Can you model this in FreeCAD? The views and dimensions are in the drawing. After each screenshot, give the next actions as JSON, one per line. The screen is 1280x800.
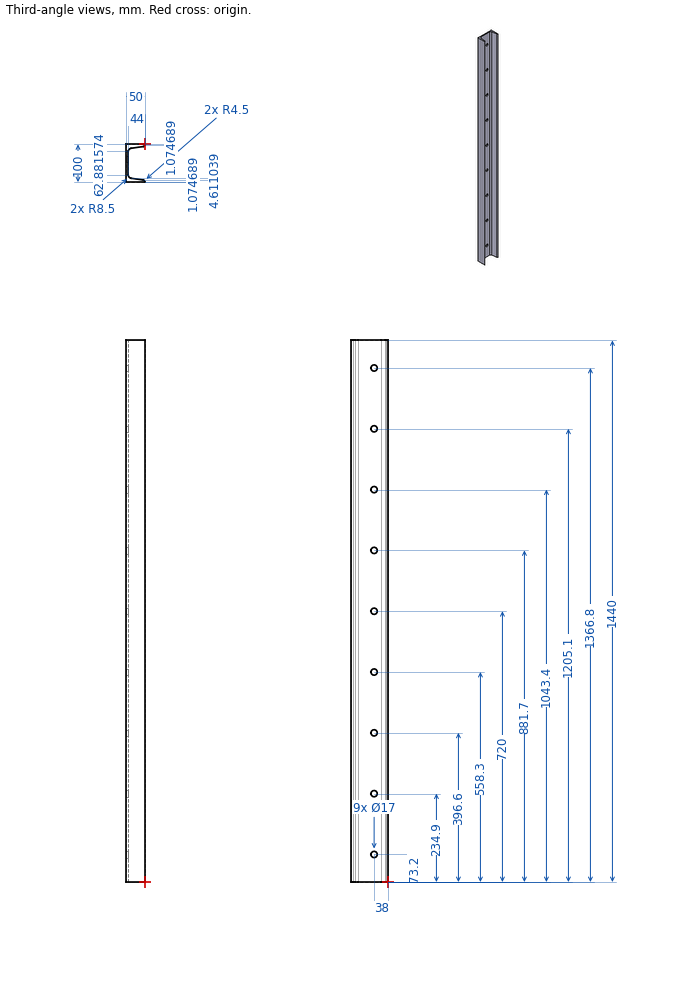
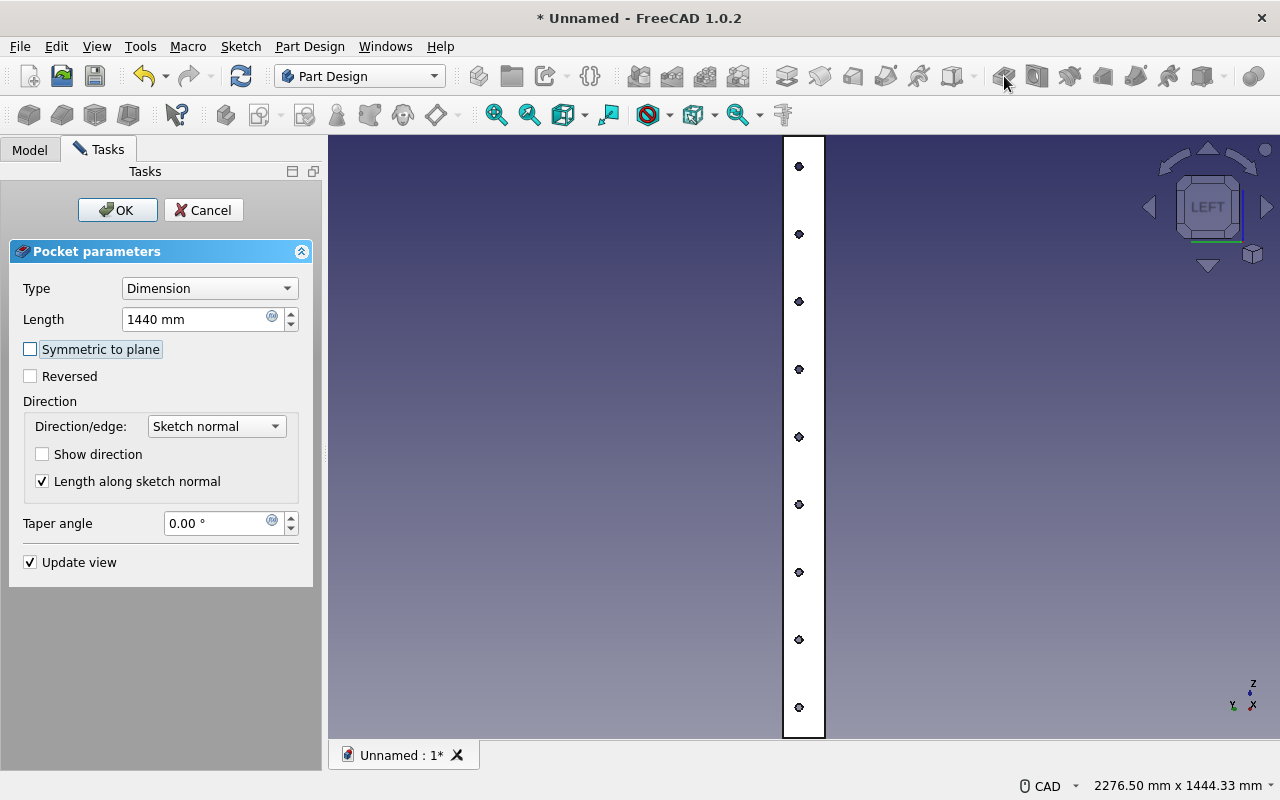
{"action": "left_click", "coordinate": [118, 210]}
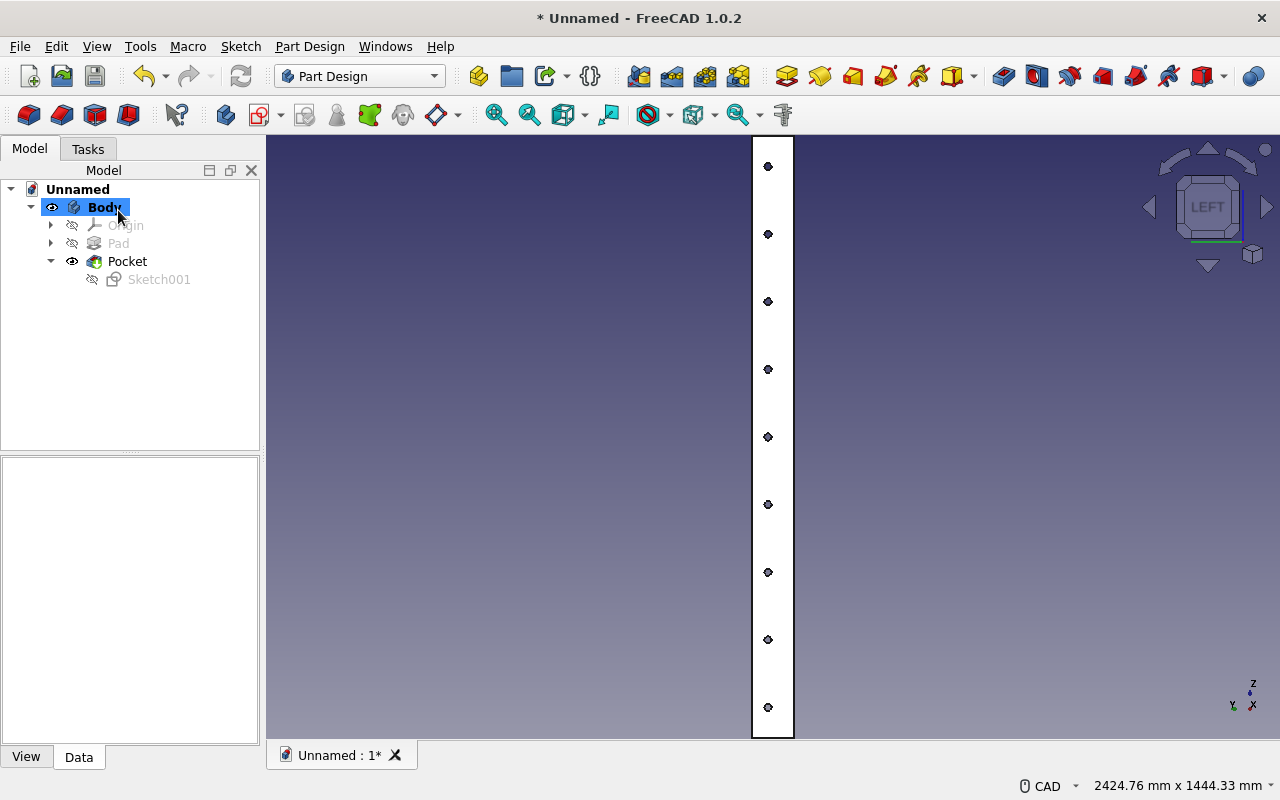
{"action": "key", "text": "0"}